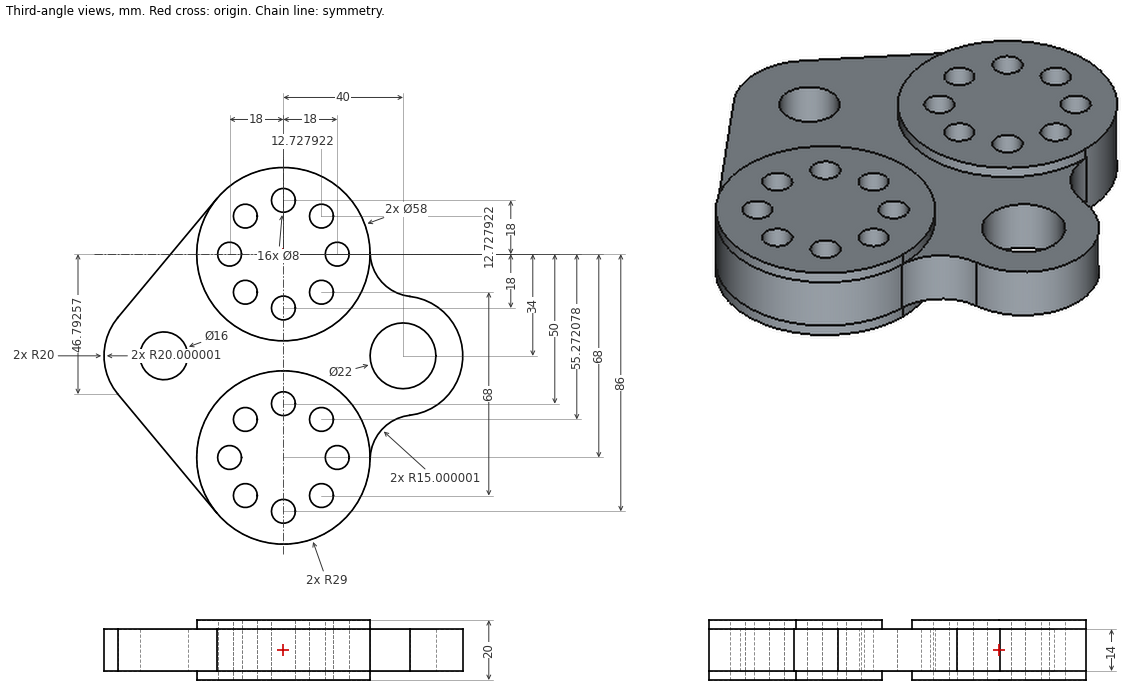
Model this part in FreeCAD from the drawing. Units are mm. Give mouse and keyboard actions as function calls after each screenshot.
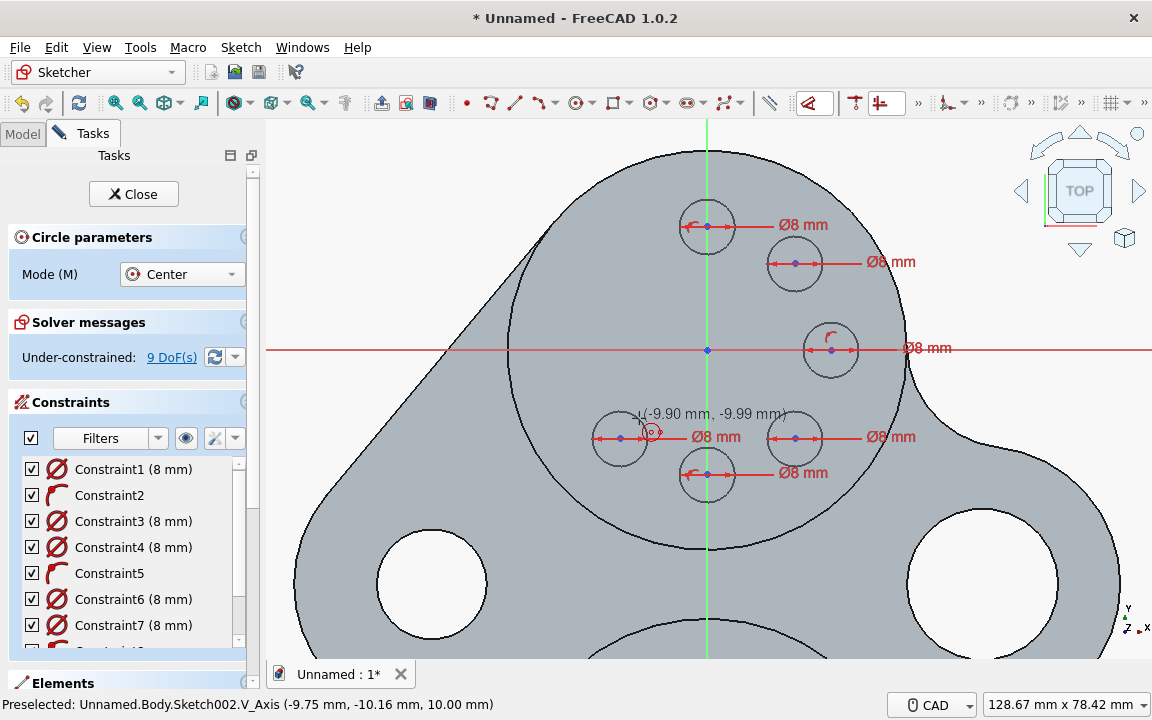
click(583, 350)
move(603, 331)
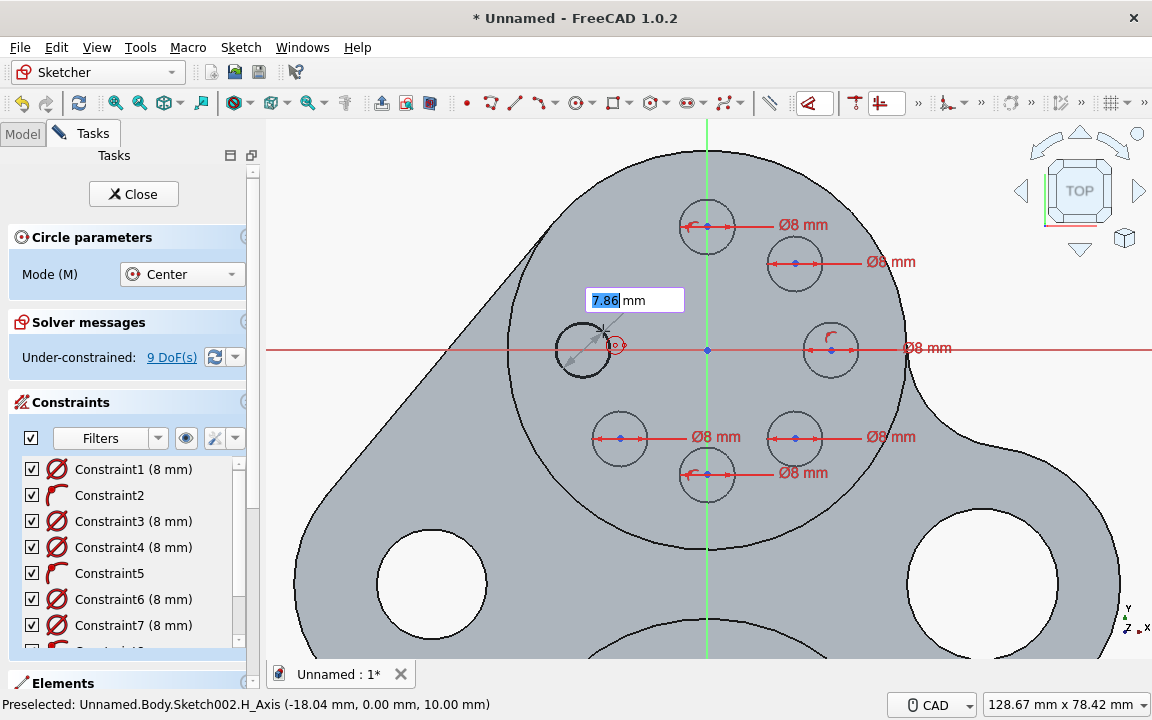
text(8)
key(Return)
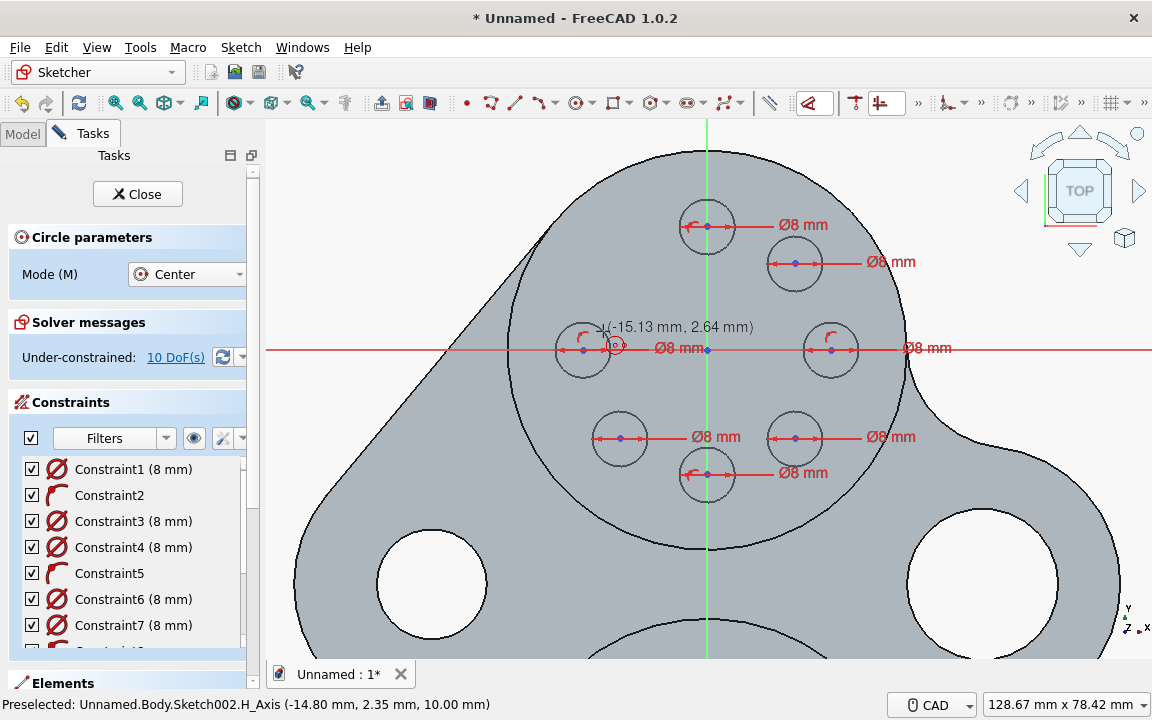
click(620, 263)
move(639, 243)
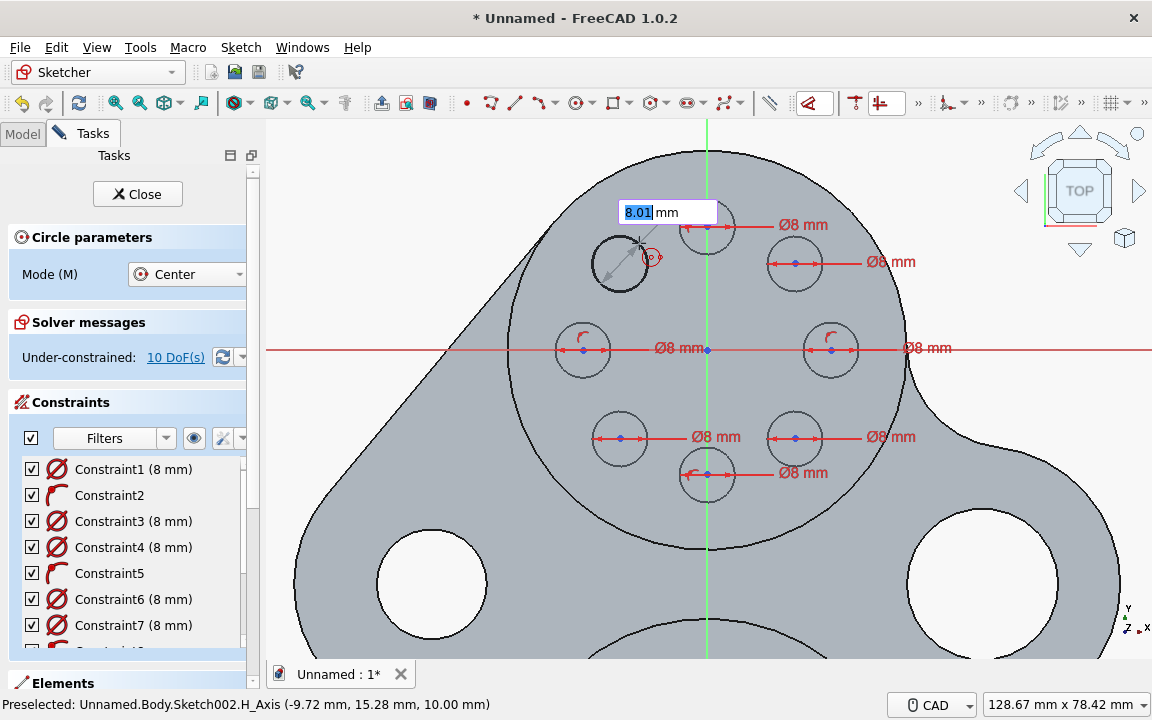
text(8)
key(Return)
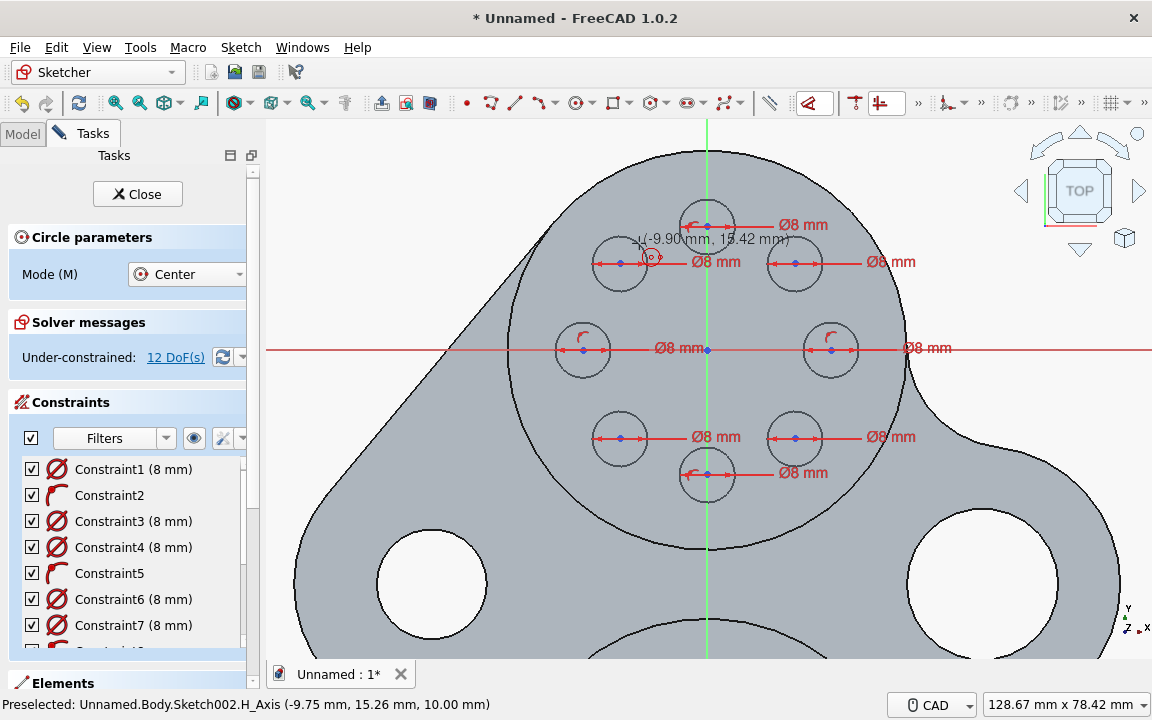
scroll(586, 230, down, 4)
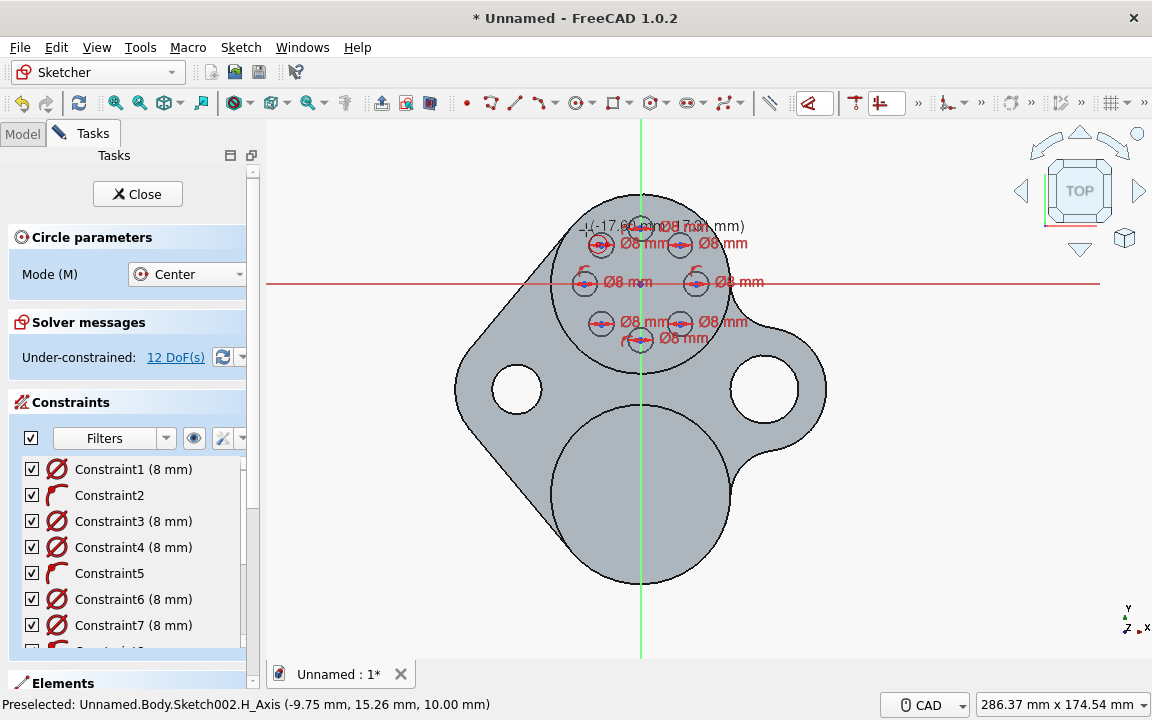
scroll(641, 439, up, 4)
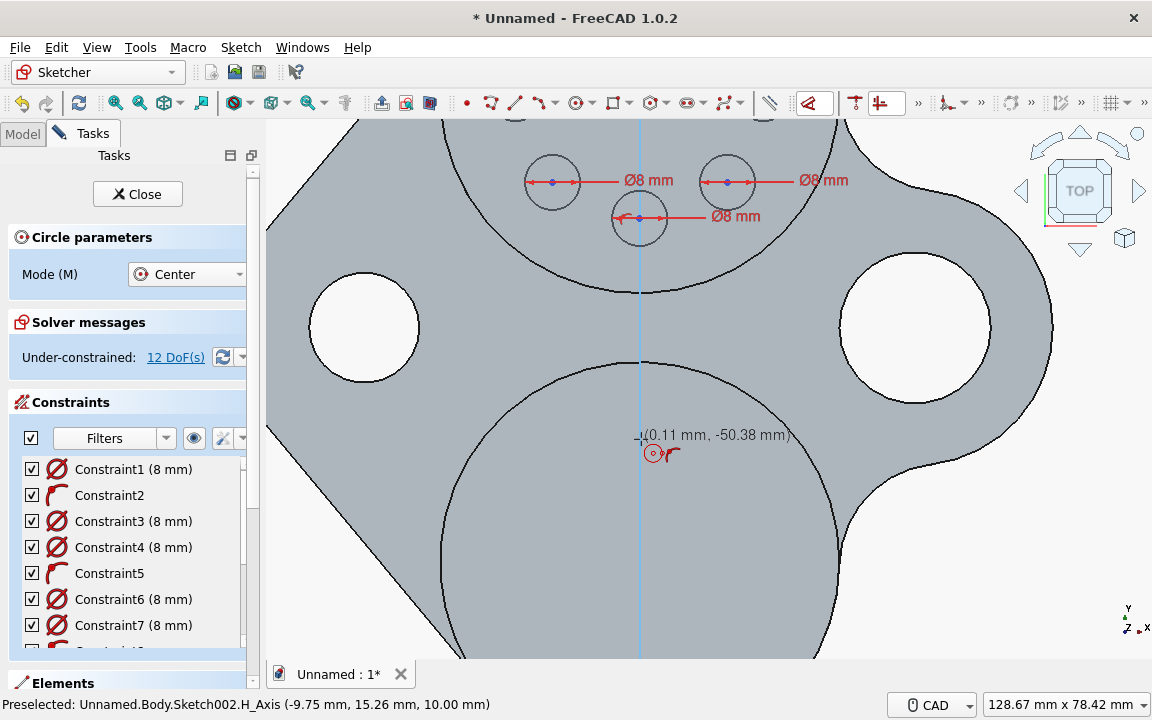
click(640, 438)
move(659, 418)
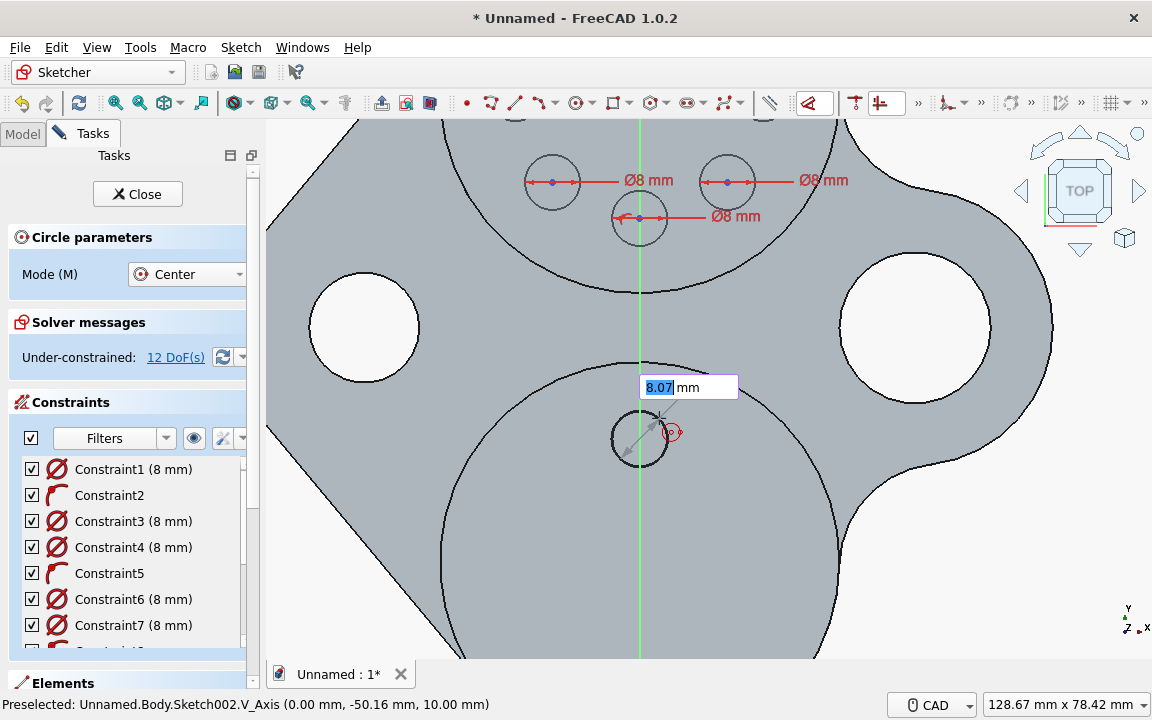
text(8)
key(Return)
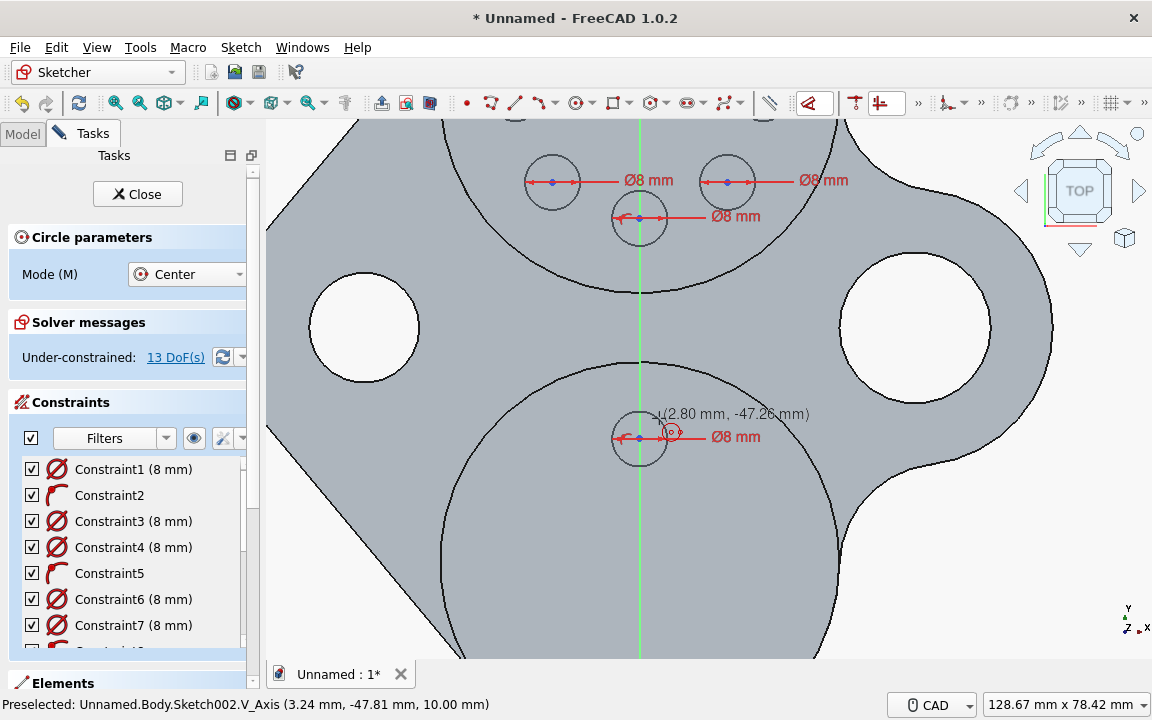
click(727, 474)
move(747, 455)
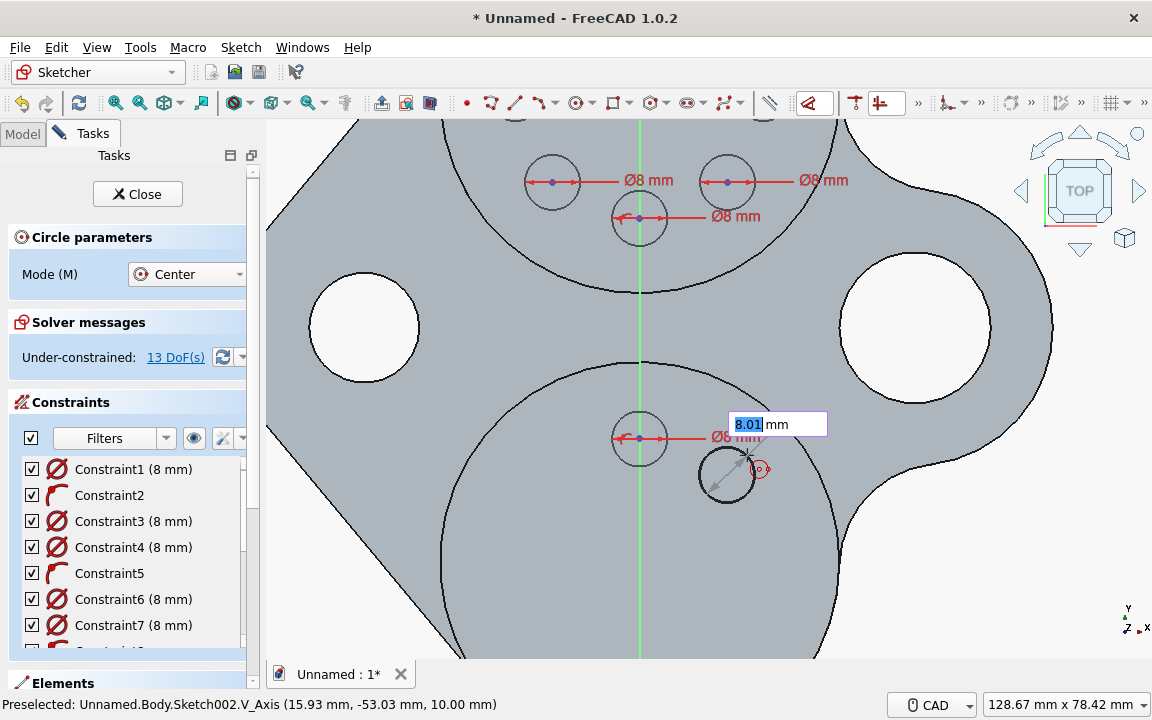
text(8)
key(Return)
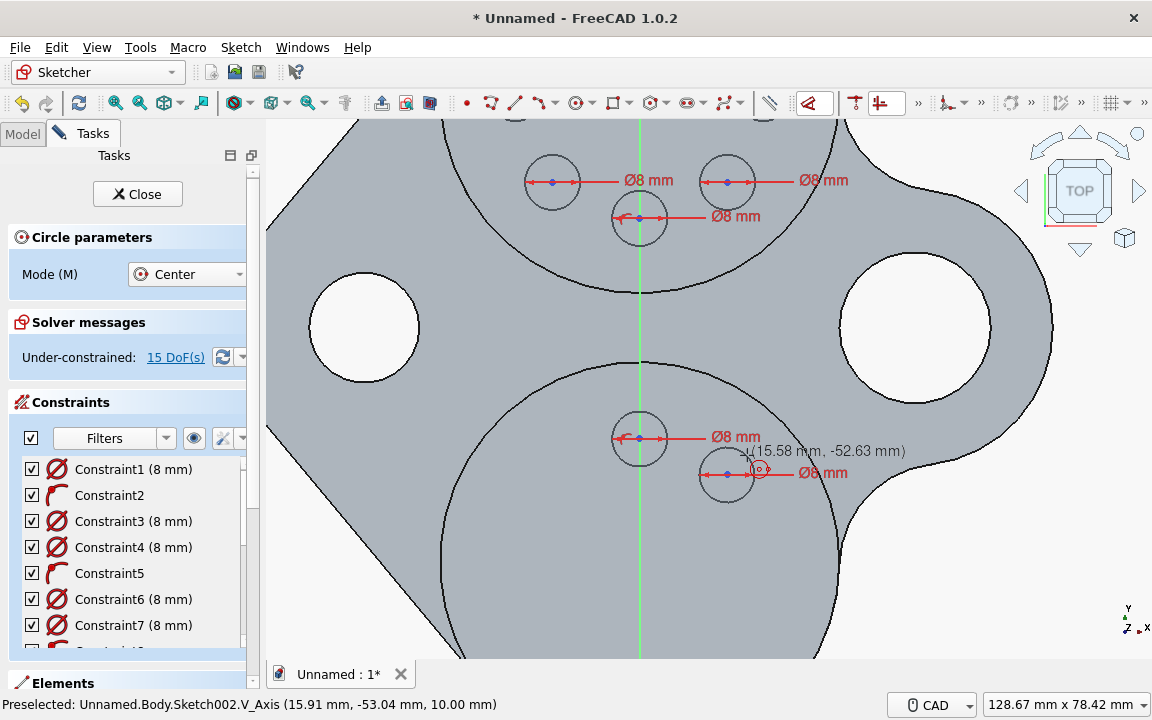
click(764, 562)
move(783, 542)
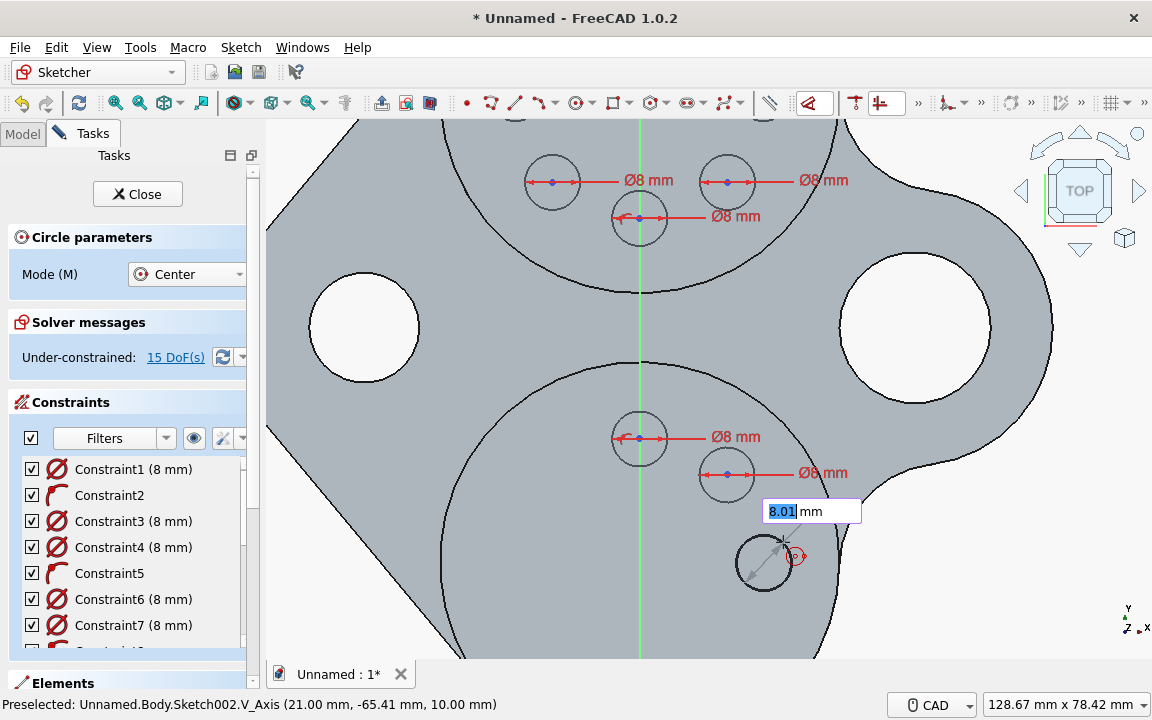
text(8)
key(Return)